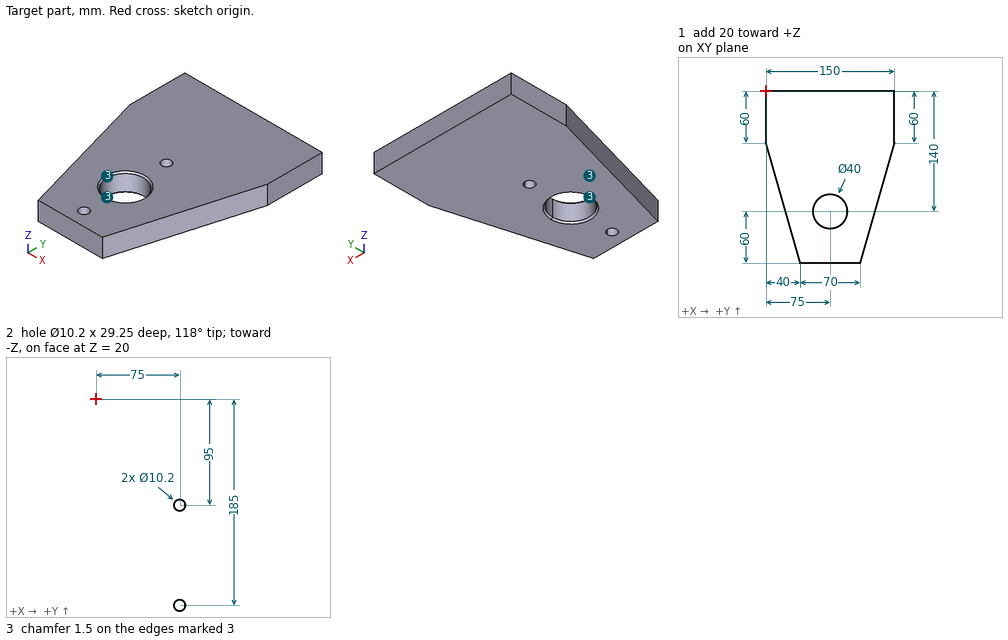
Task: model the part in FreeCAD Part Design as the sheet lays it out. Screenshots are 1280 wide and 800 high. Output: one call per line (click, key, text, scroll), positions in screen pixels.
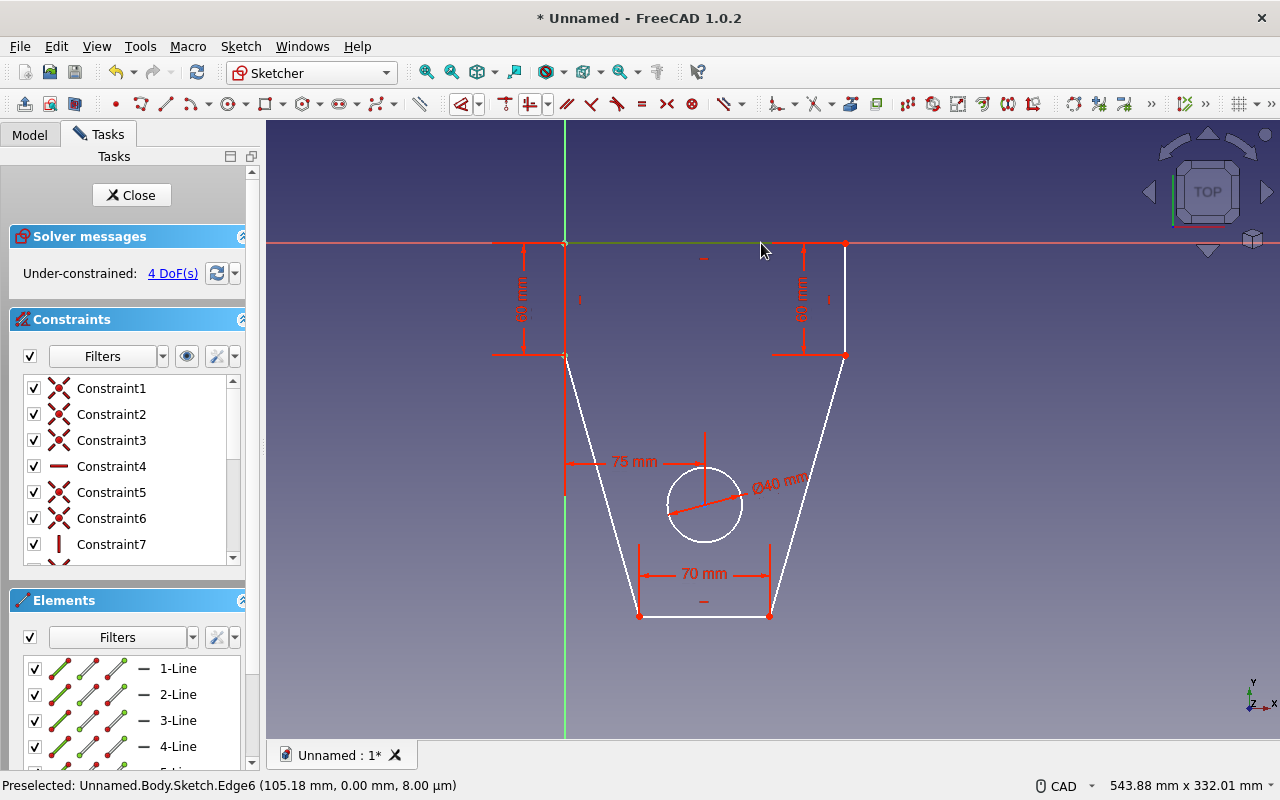
click(478, 104)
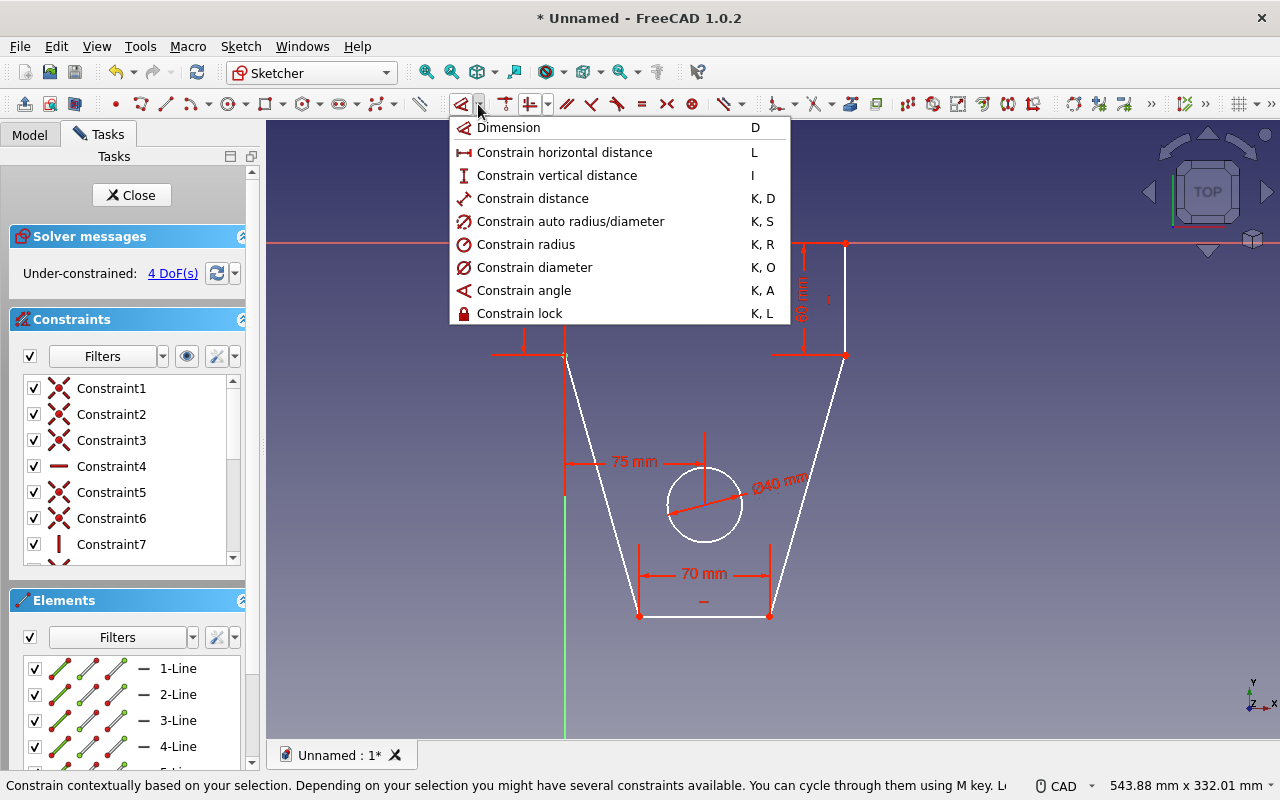
click(620, 152)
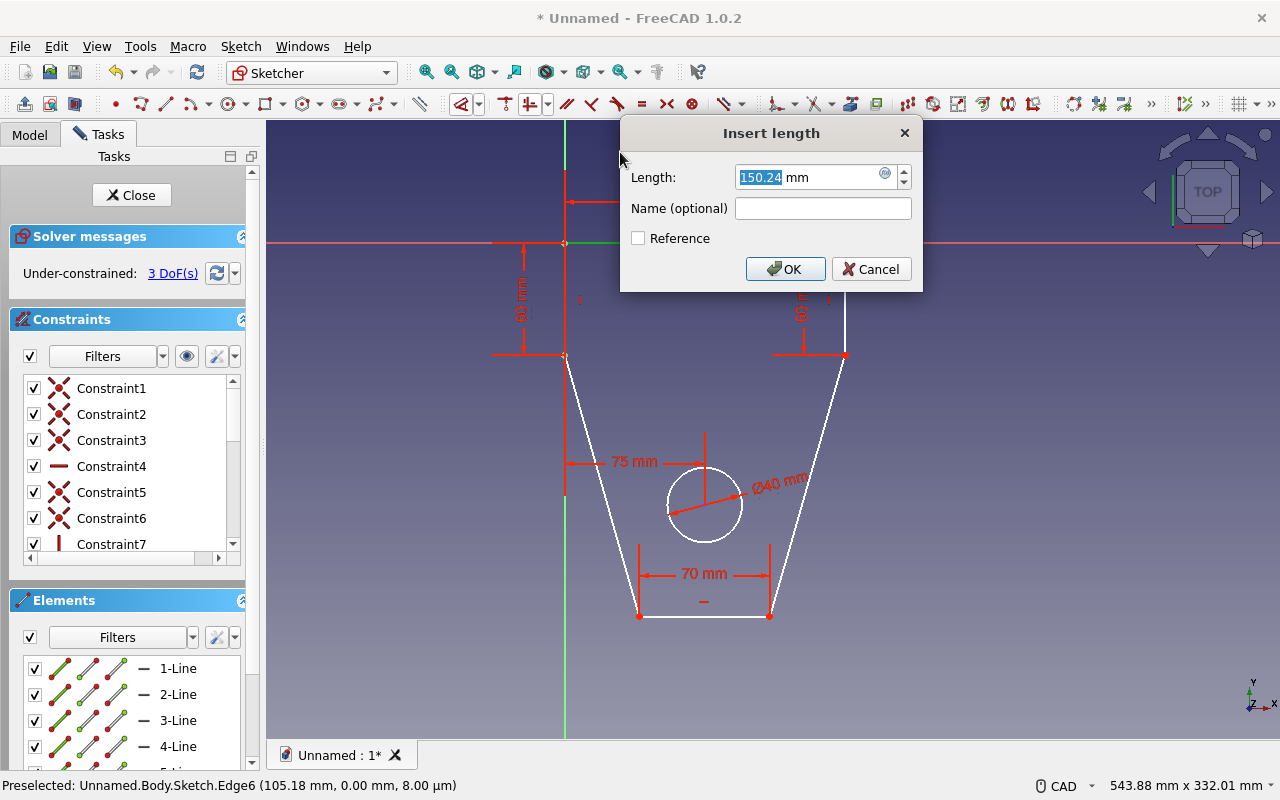
text(150)
key(Return)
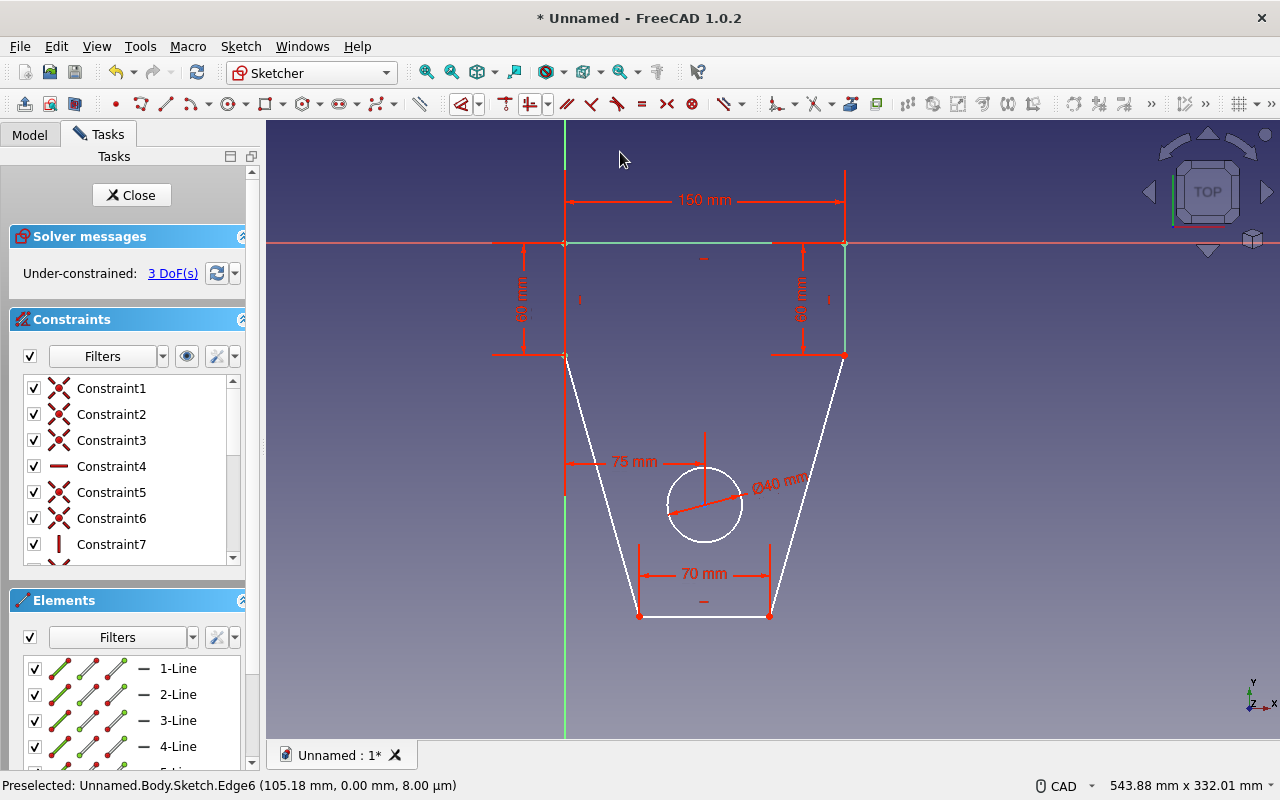
click(639, 617)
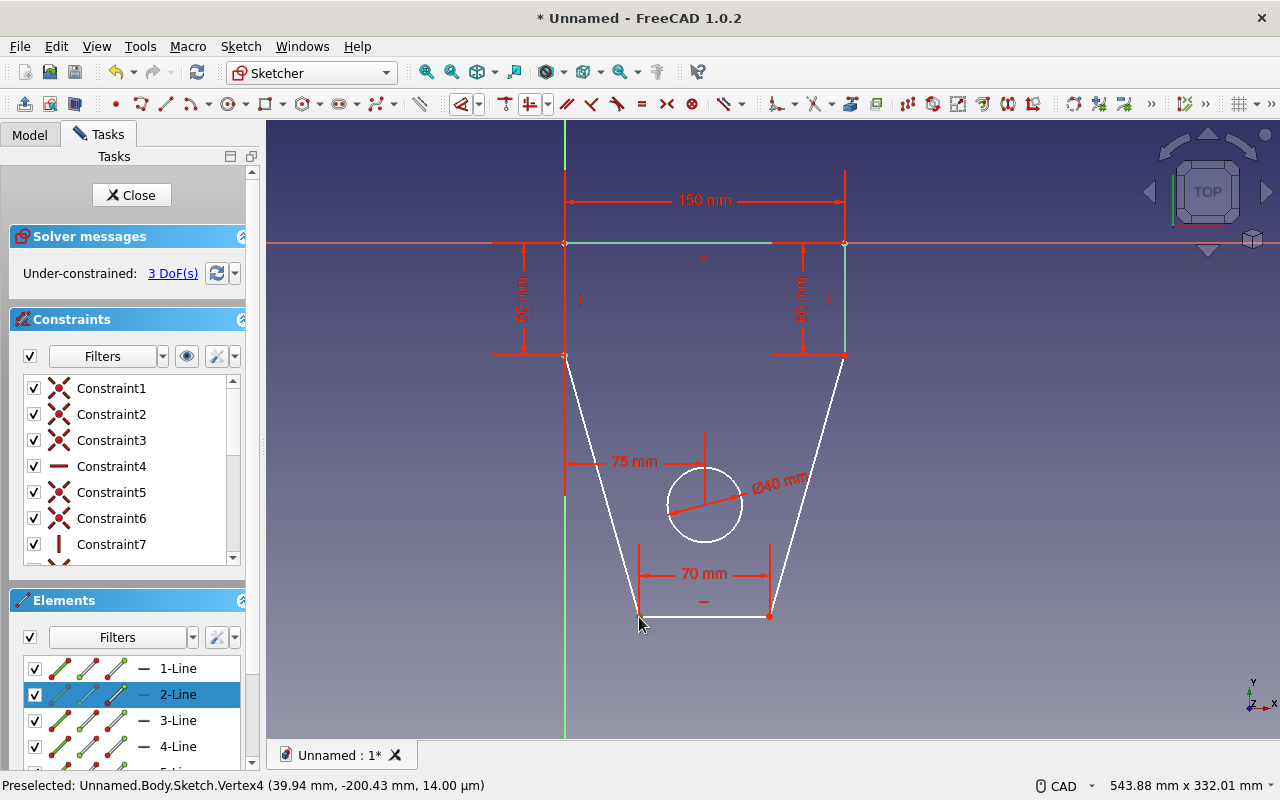
key(l)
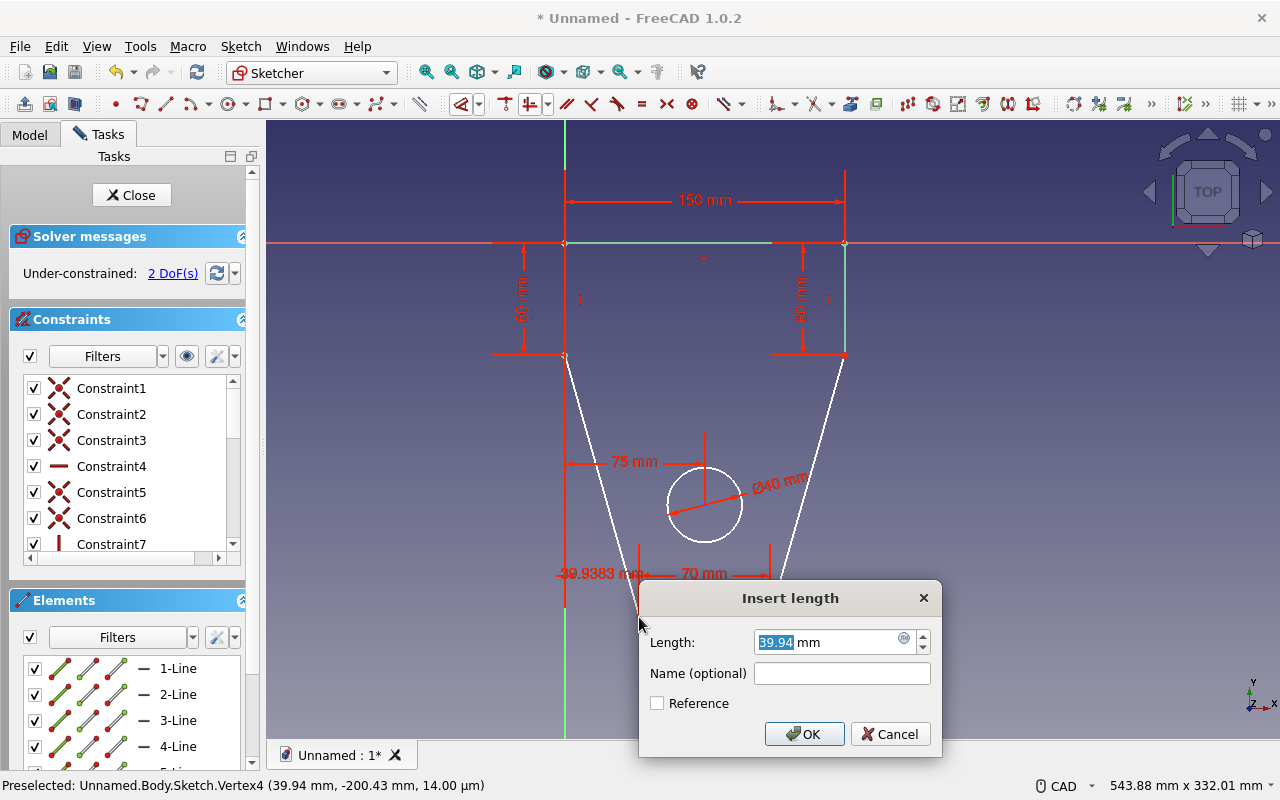
text(40)
key(Return)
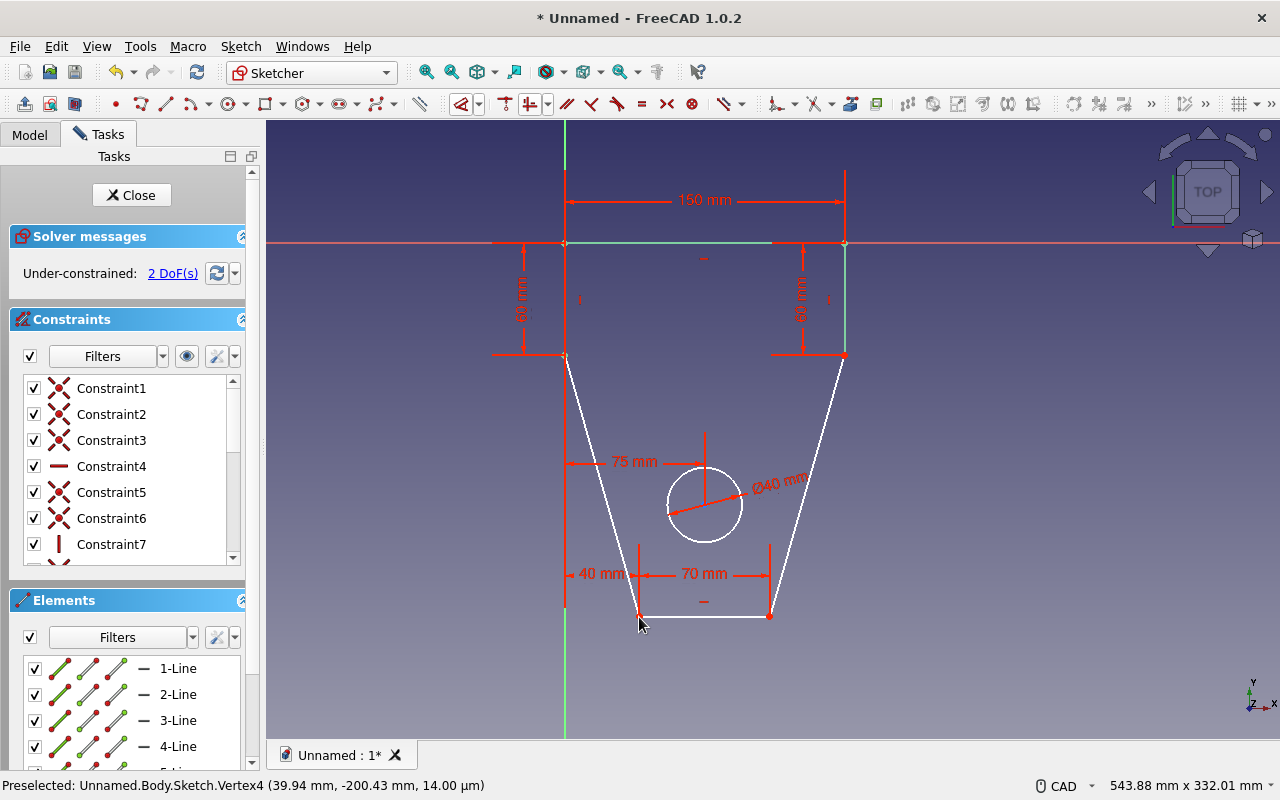
click(705, 505)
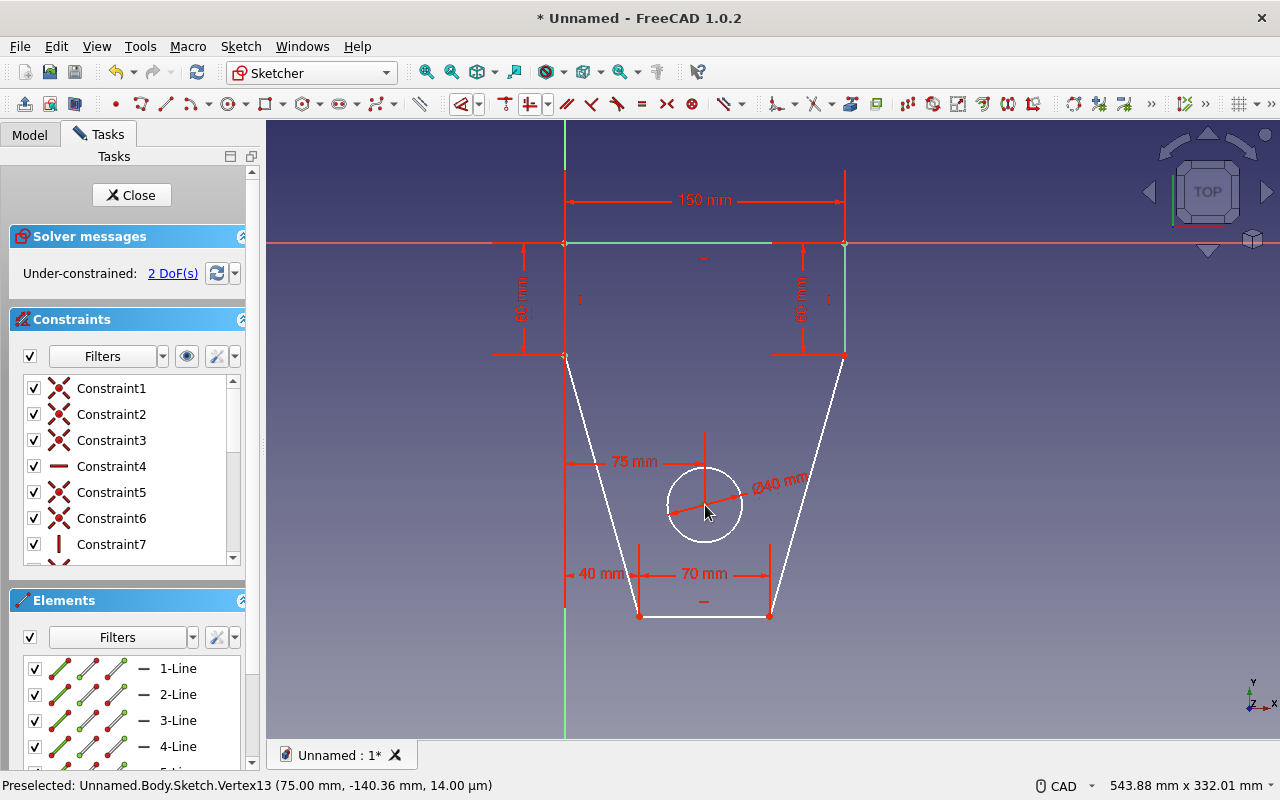
key(i)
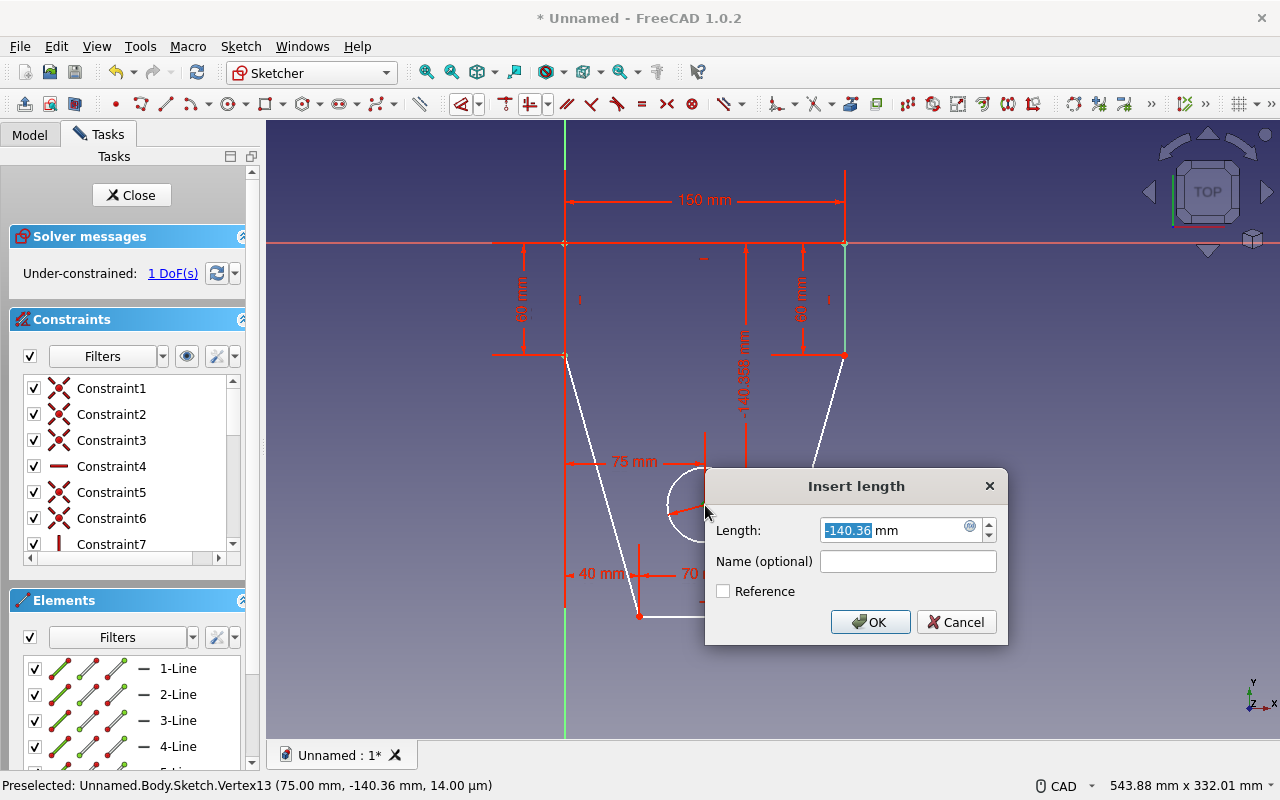
text(-140)
key(Return)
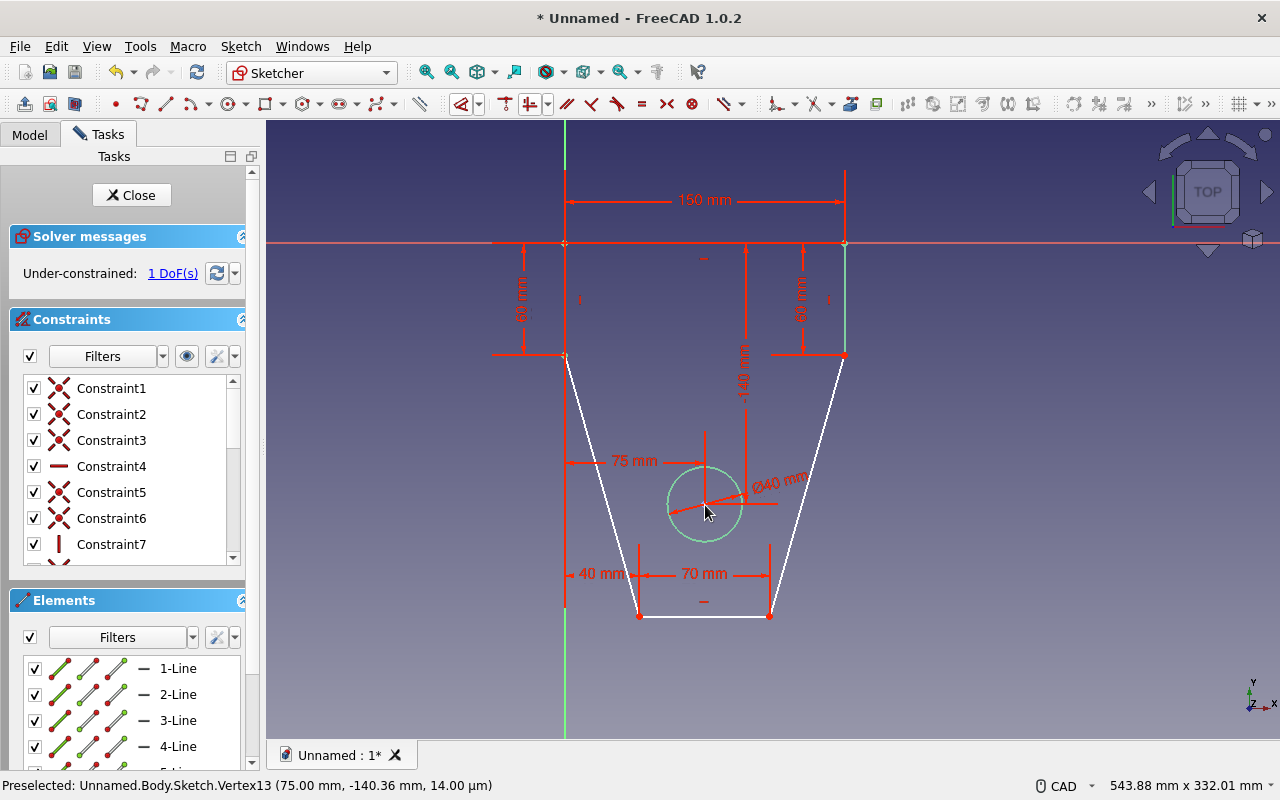
click(639, 617)